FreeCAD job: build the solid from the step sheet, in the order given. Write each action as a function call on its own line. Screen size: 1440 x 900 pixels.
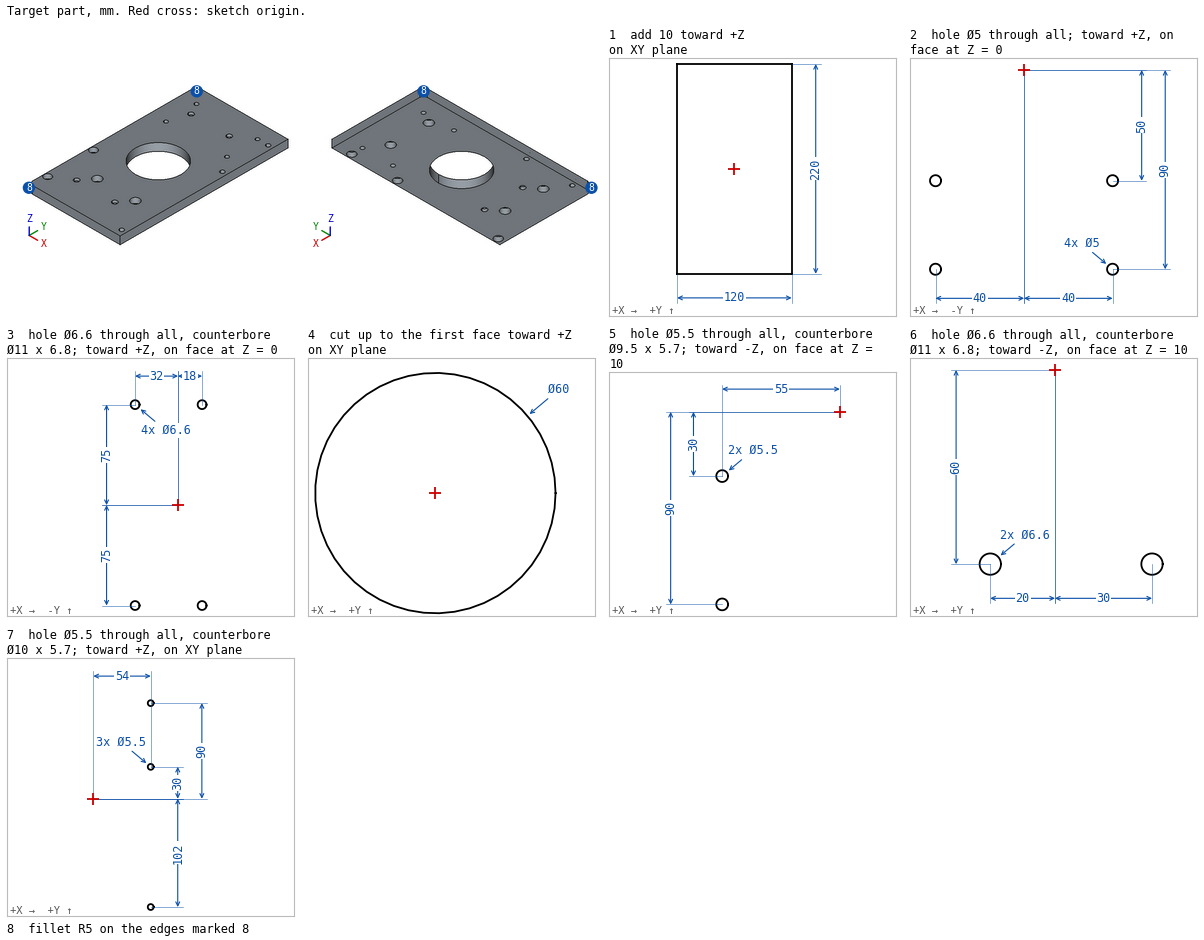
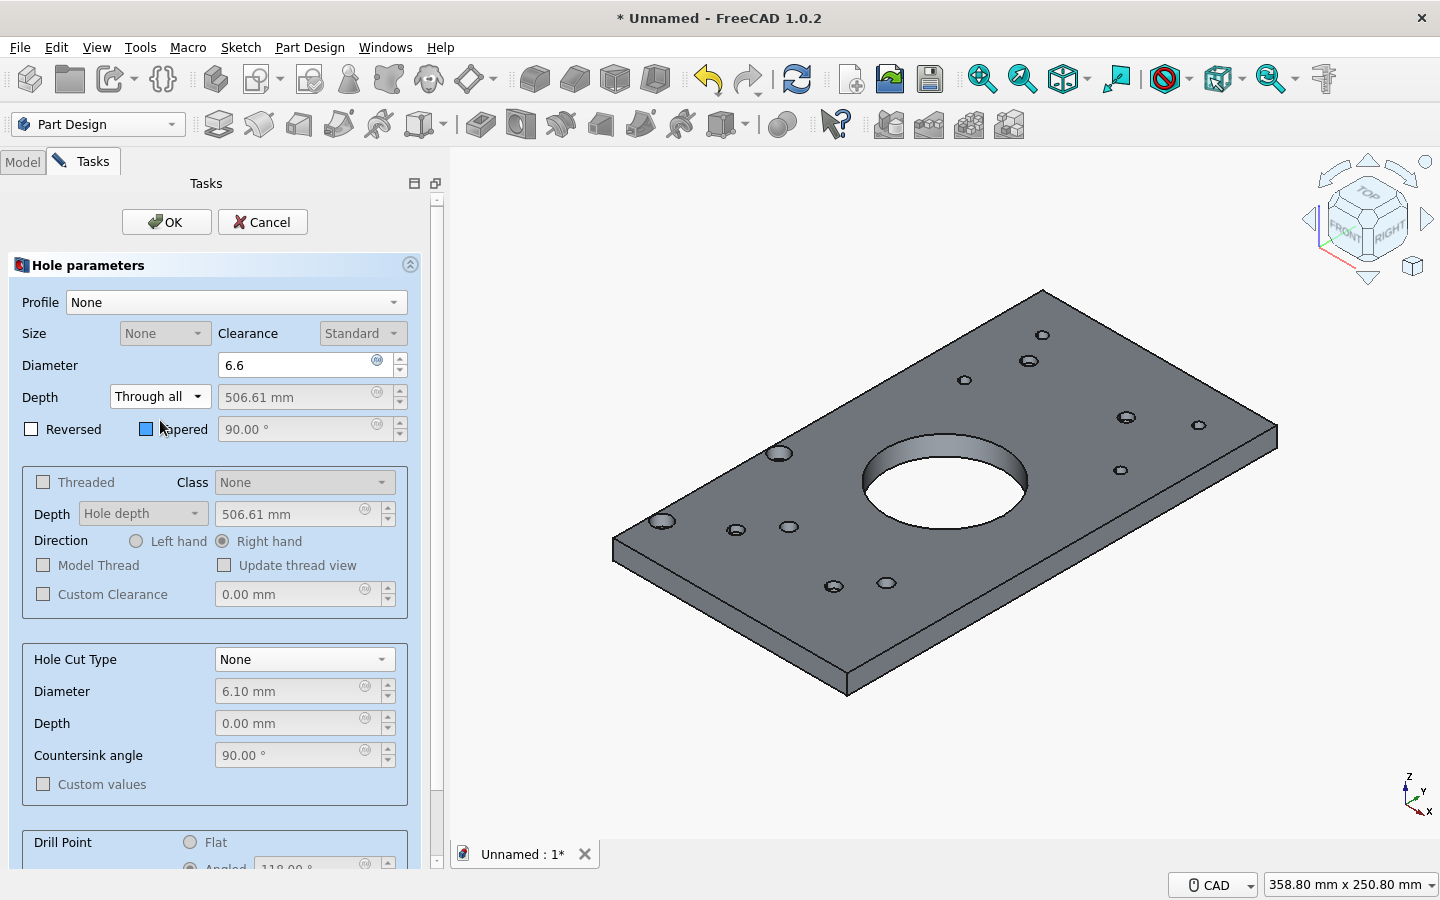
click(306, 660)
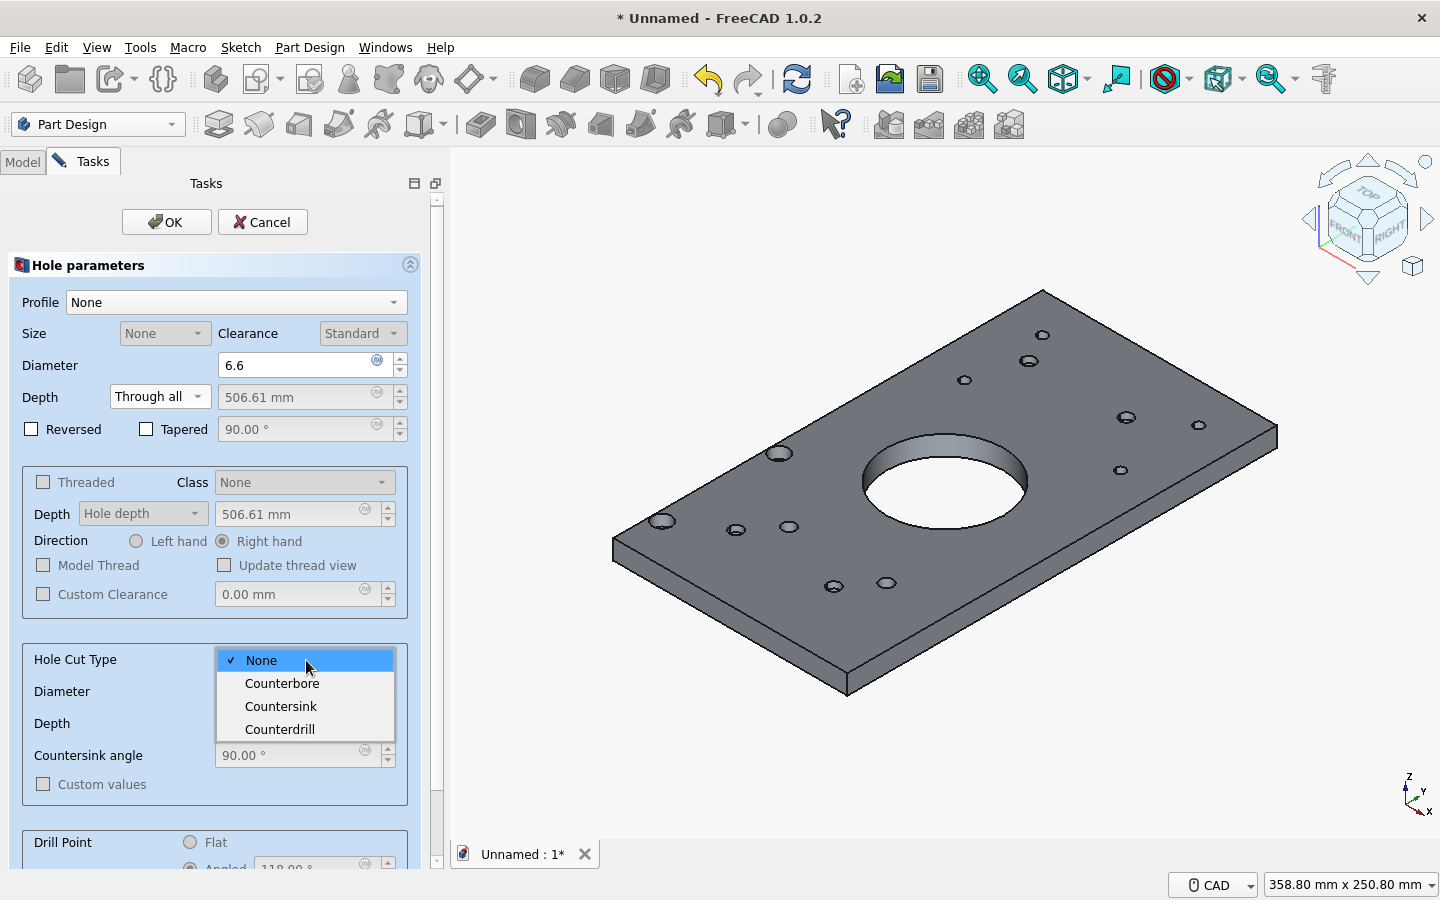
click(304, 684)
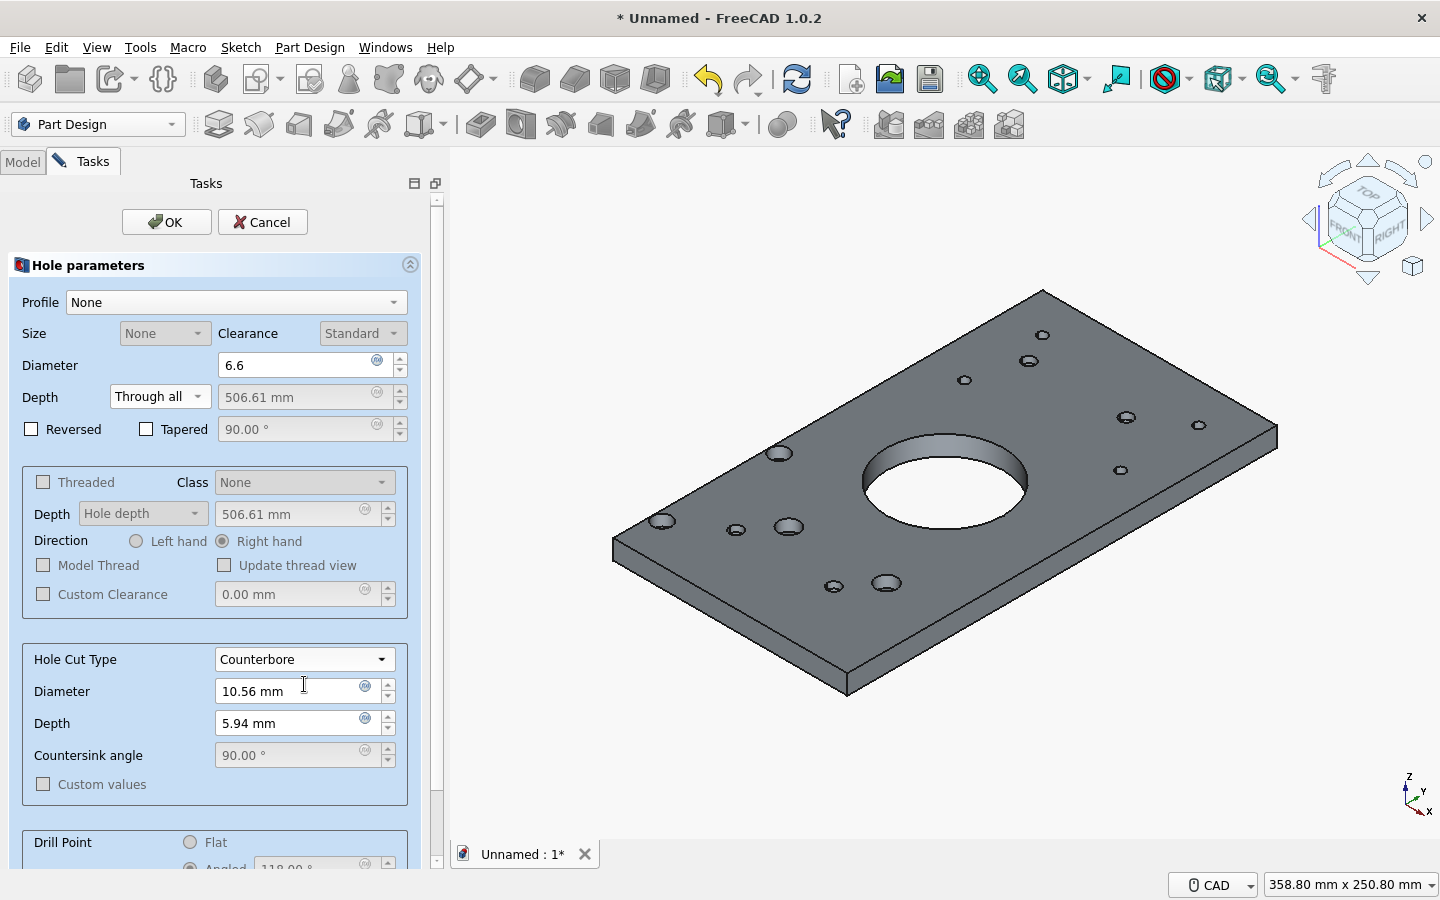
triple_click(298, 691)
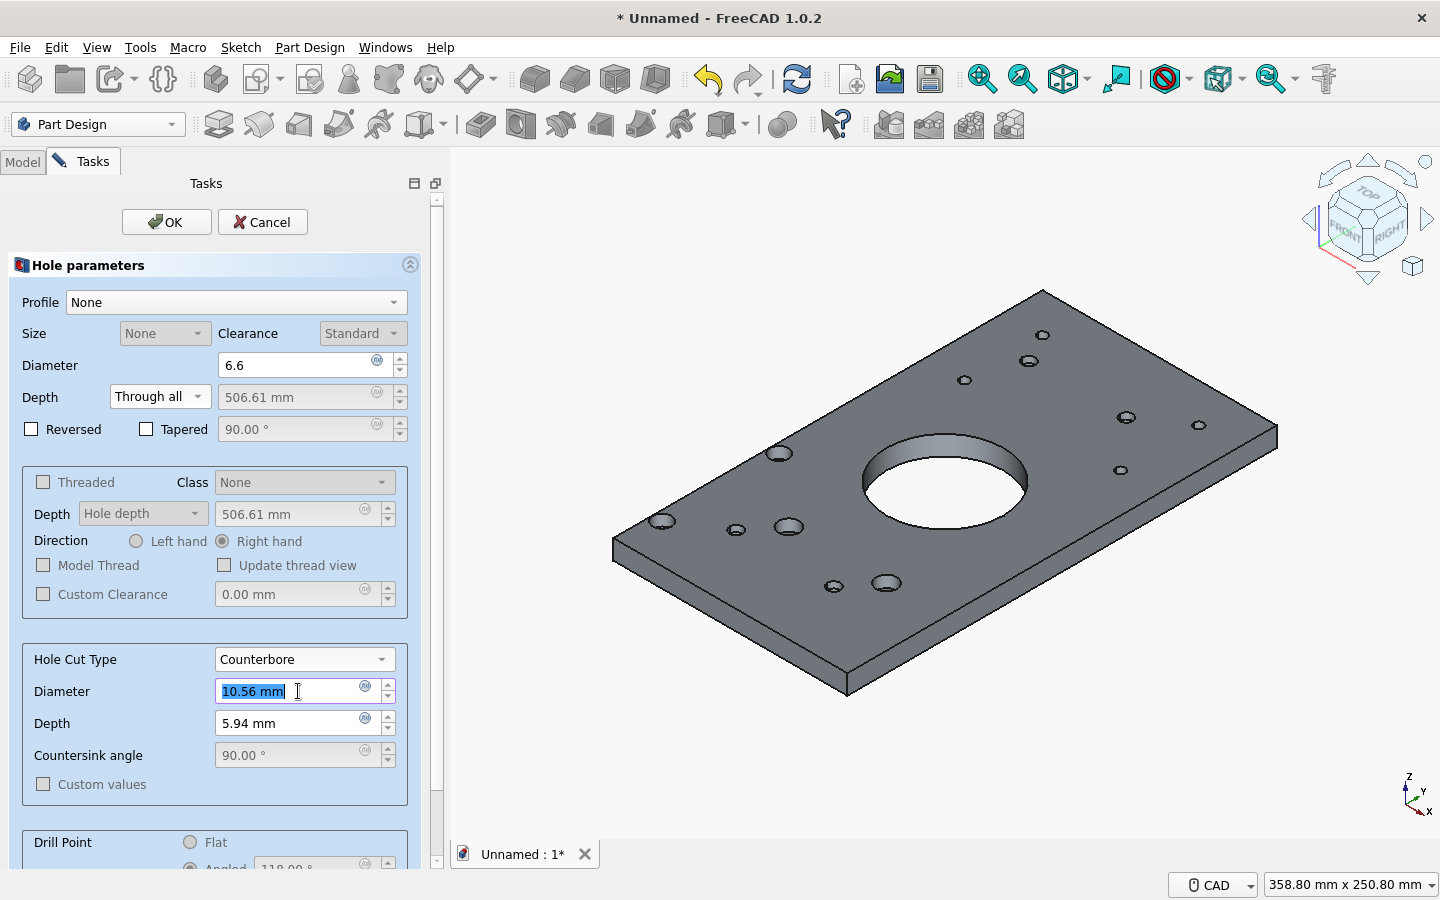
text(11)
key(Tab)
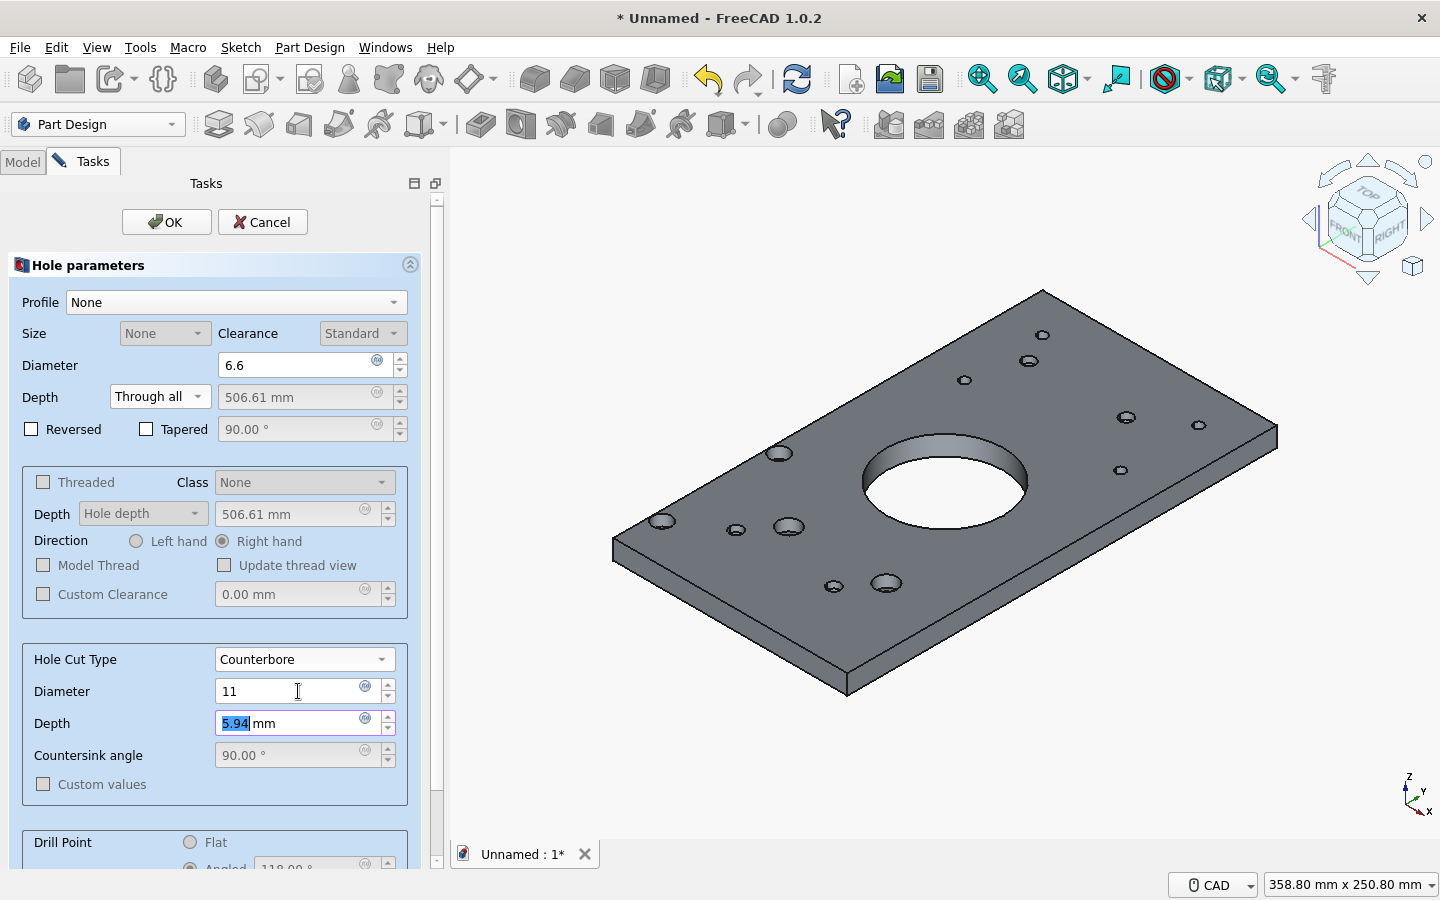
text(6.8)
key(Tab)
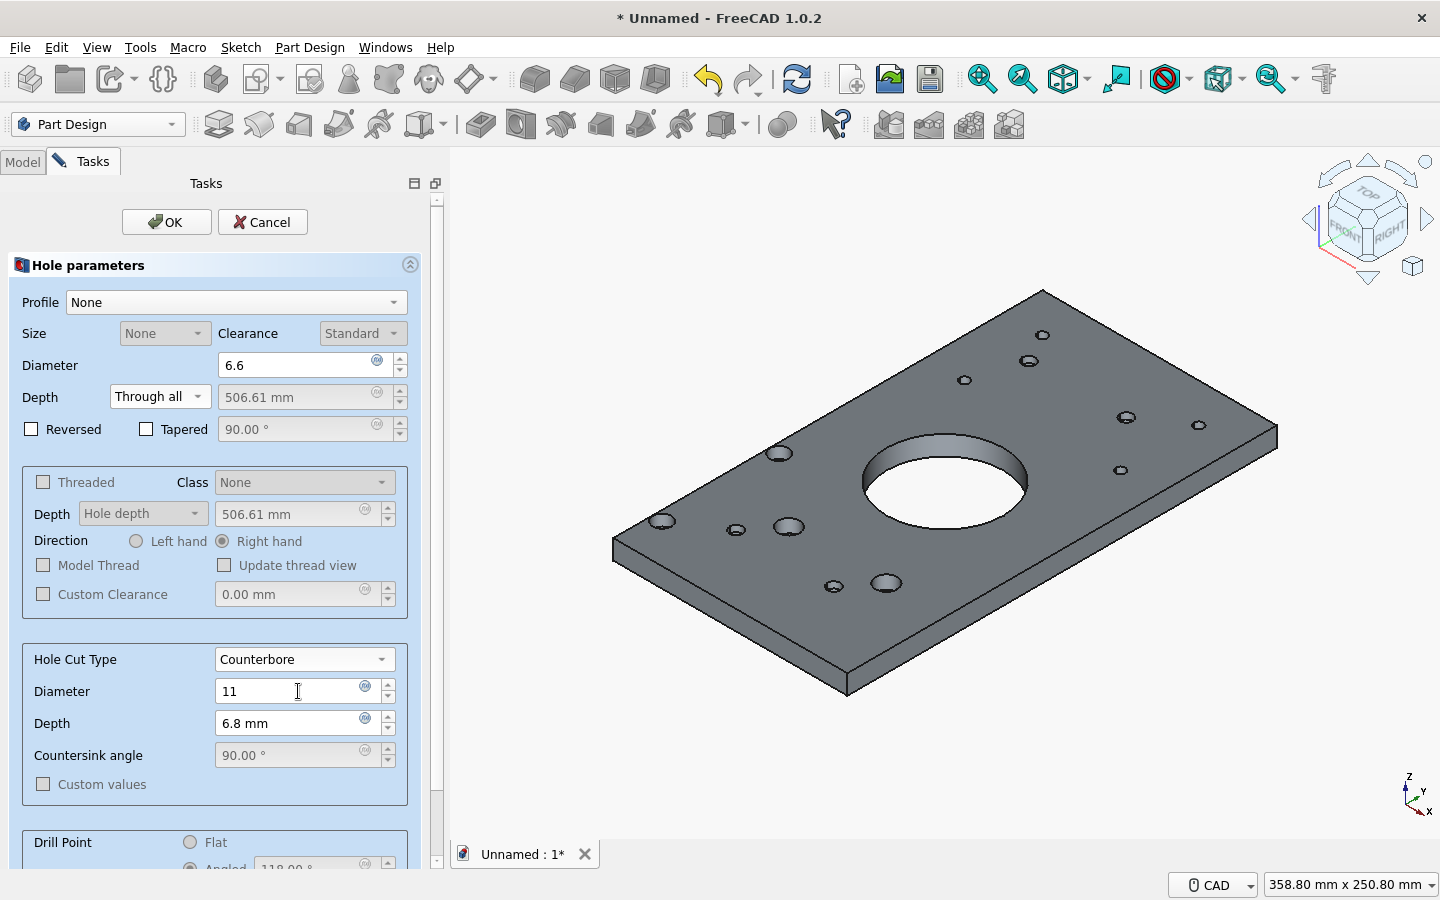
click(167, 222)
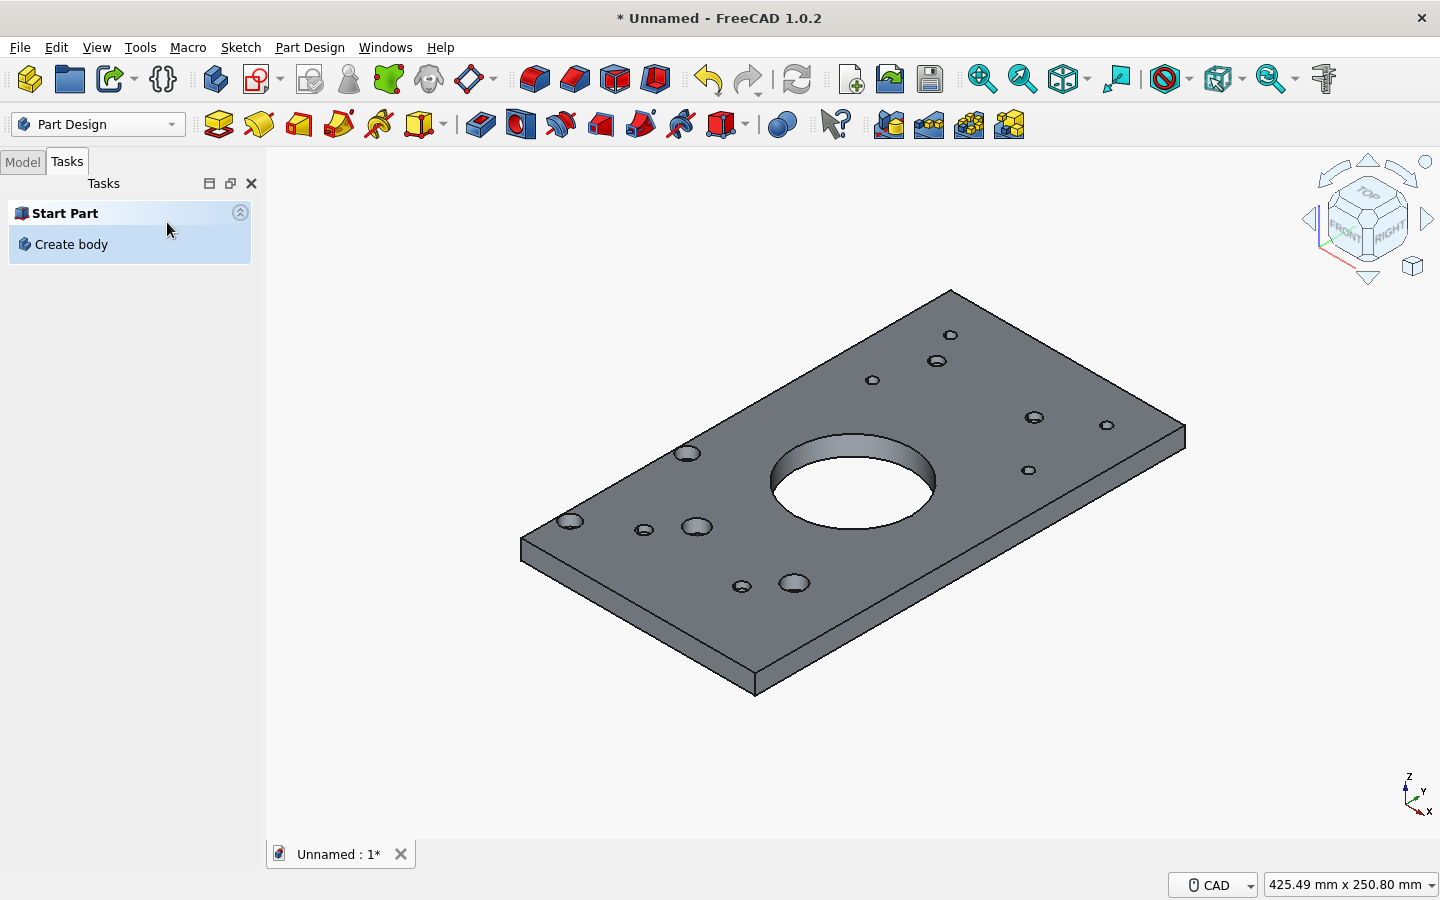
click(256, 80)